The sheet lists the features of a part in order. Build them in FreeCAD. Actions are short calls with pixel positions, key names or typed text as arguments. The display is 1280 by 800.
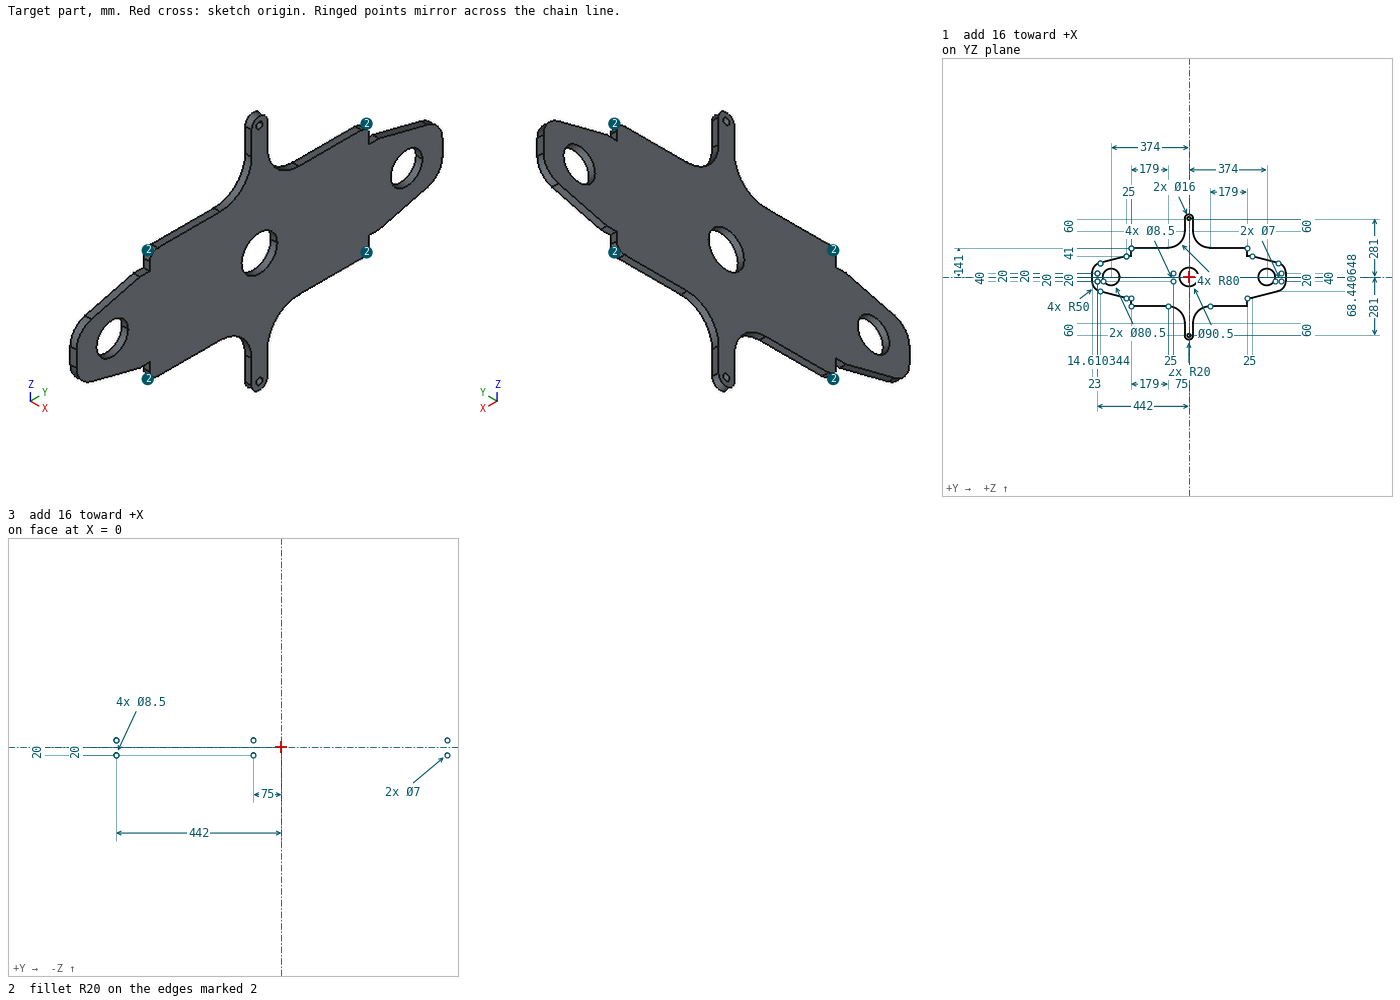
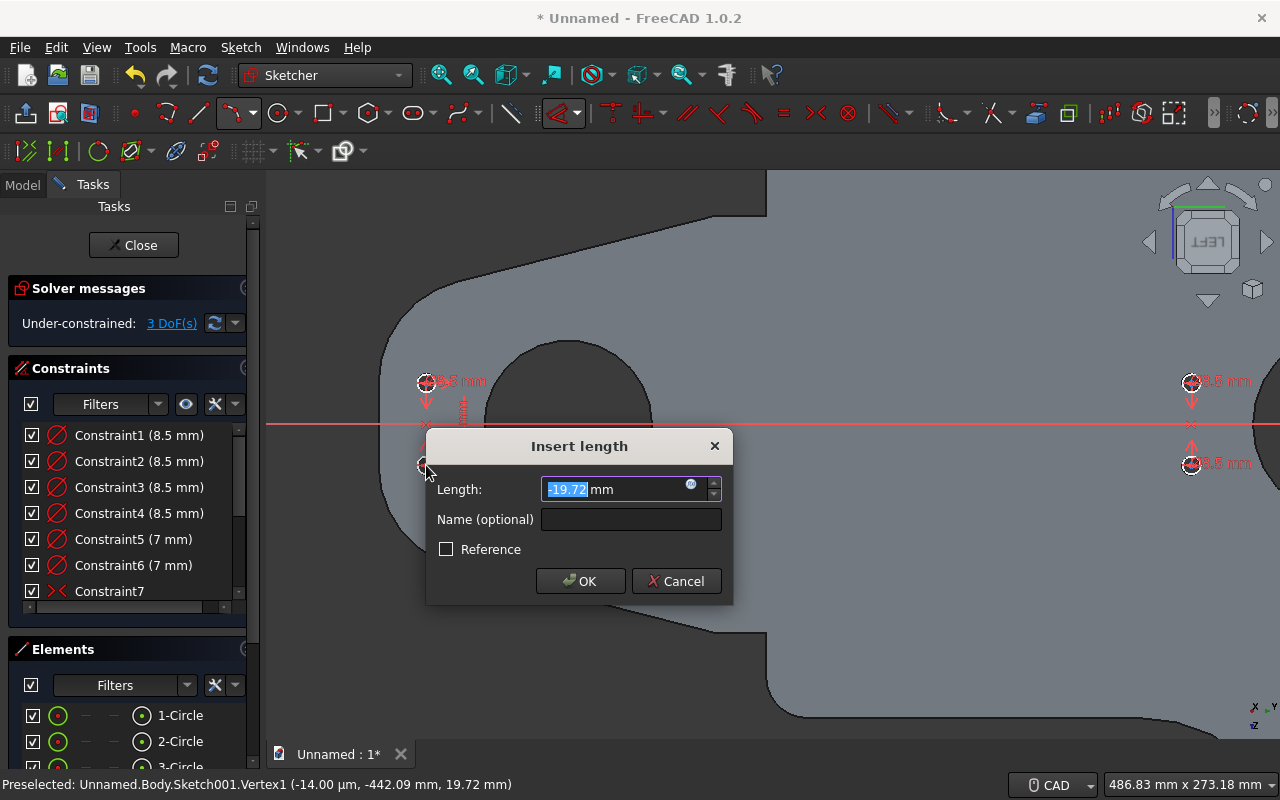
text(-20)
key(Return)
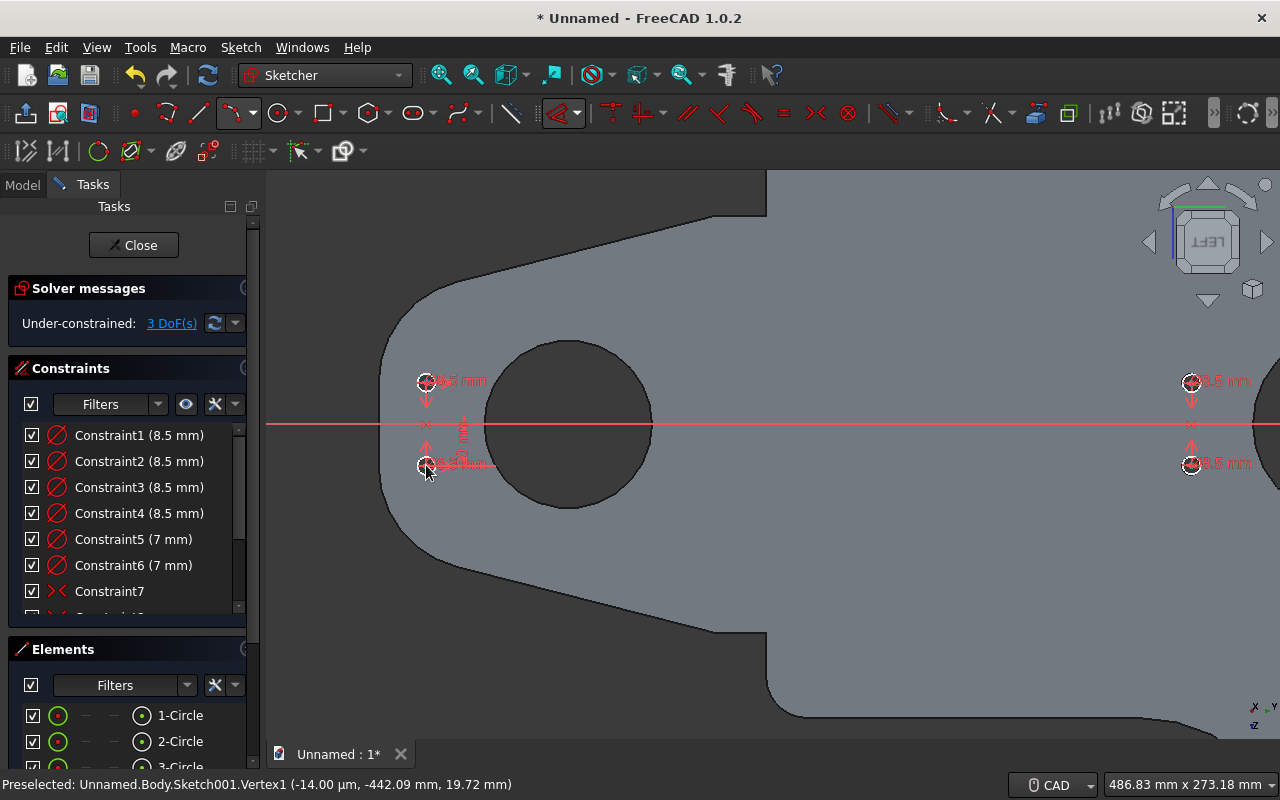
scroll(428, 467, down, 6)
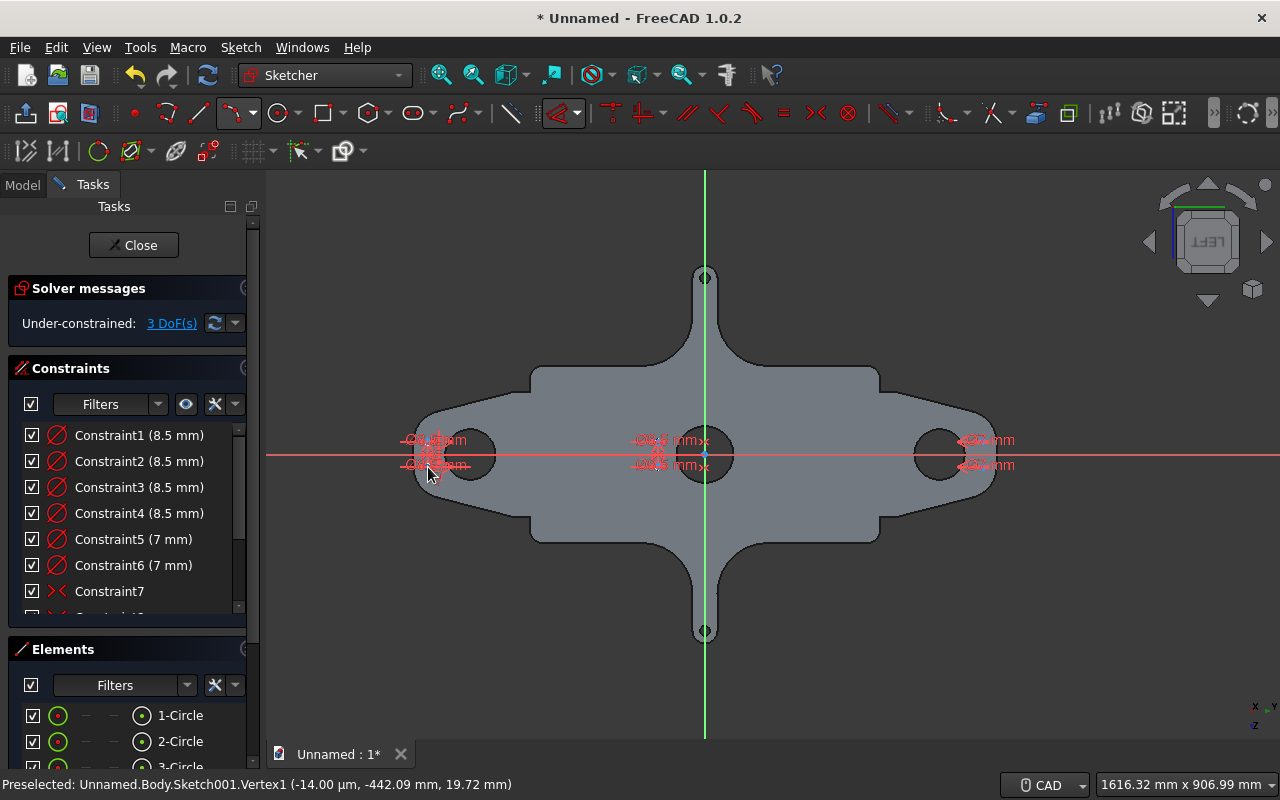
click(658, 467)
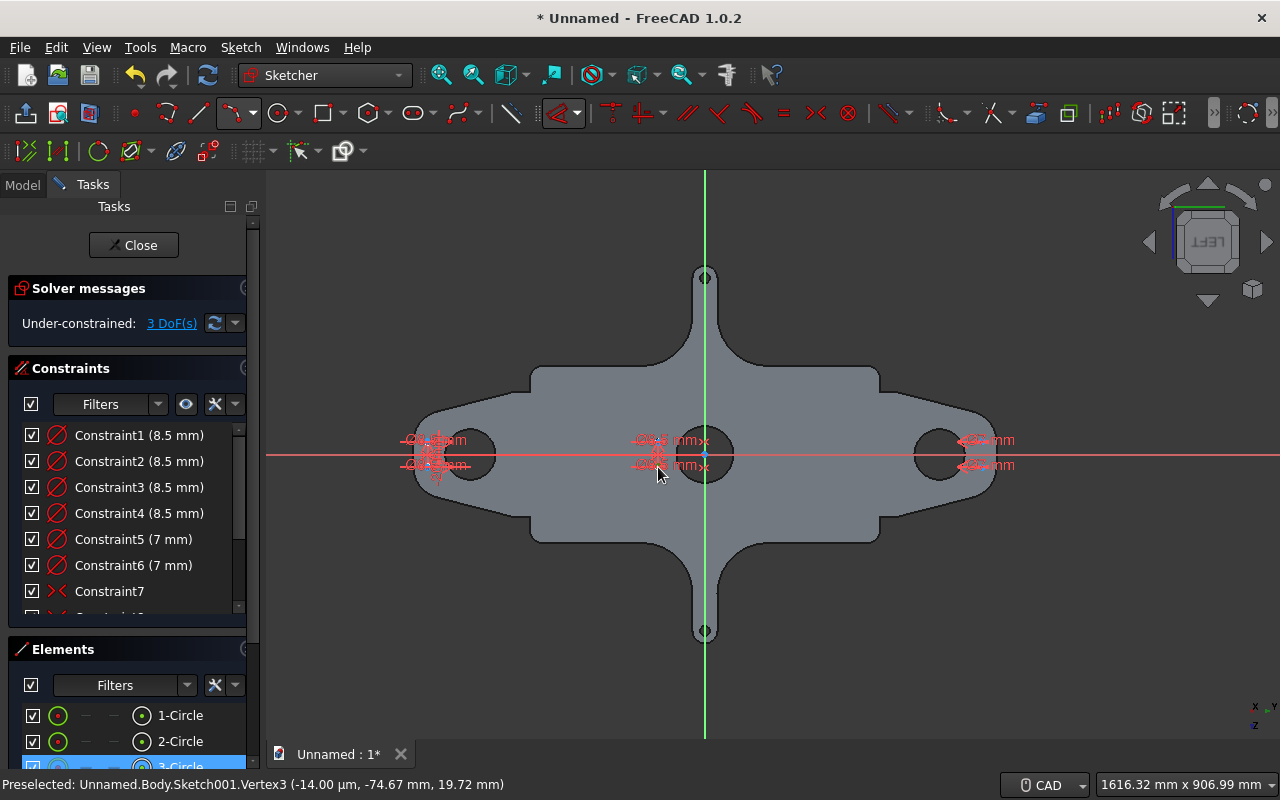
key(l)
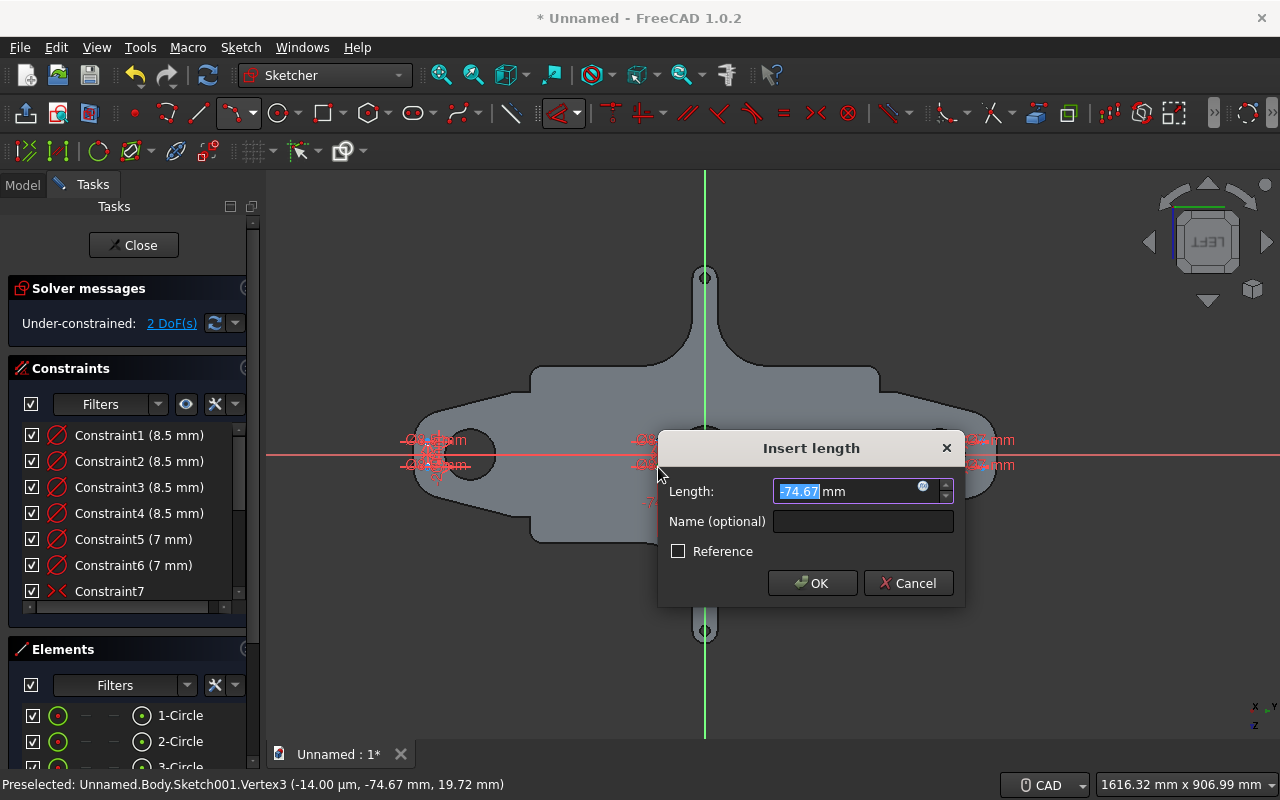
text(-75)
key(Return)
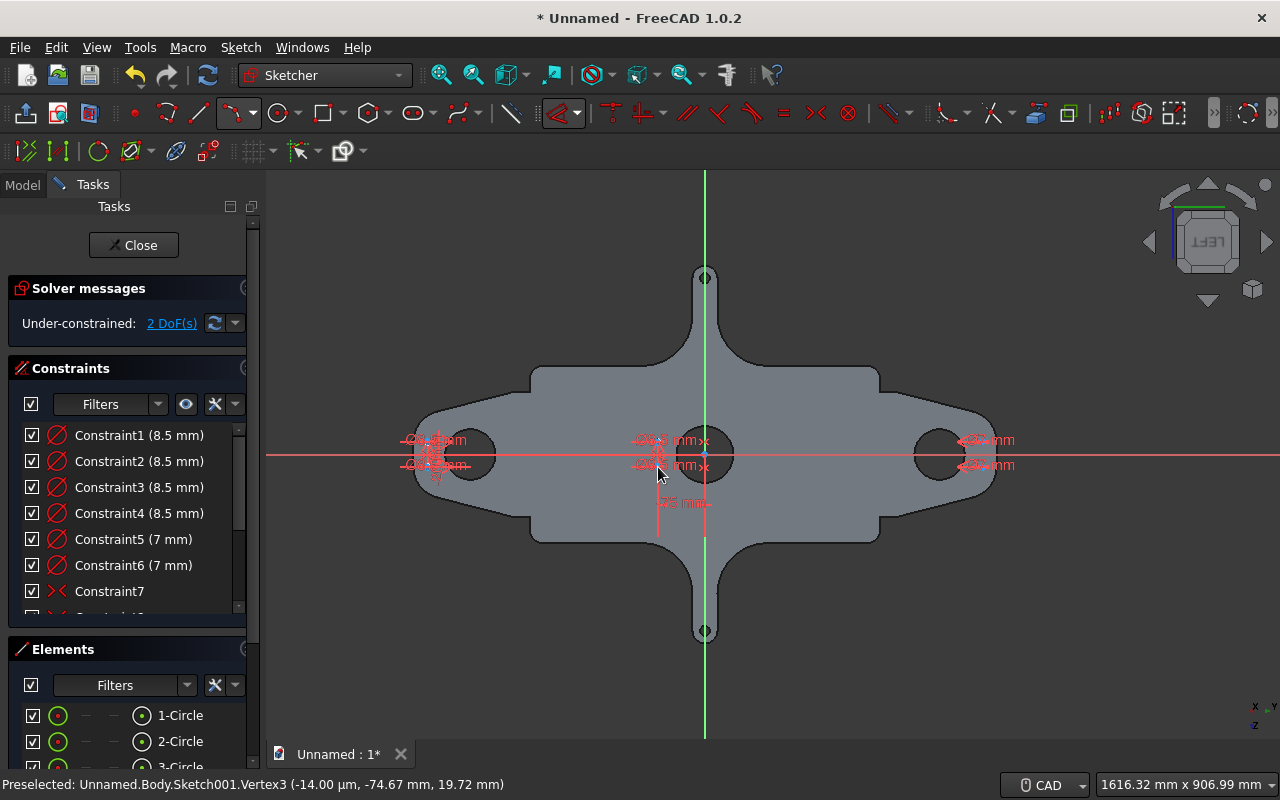
scroll(658, 467, up, 6)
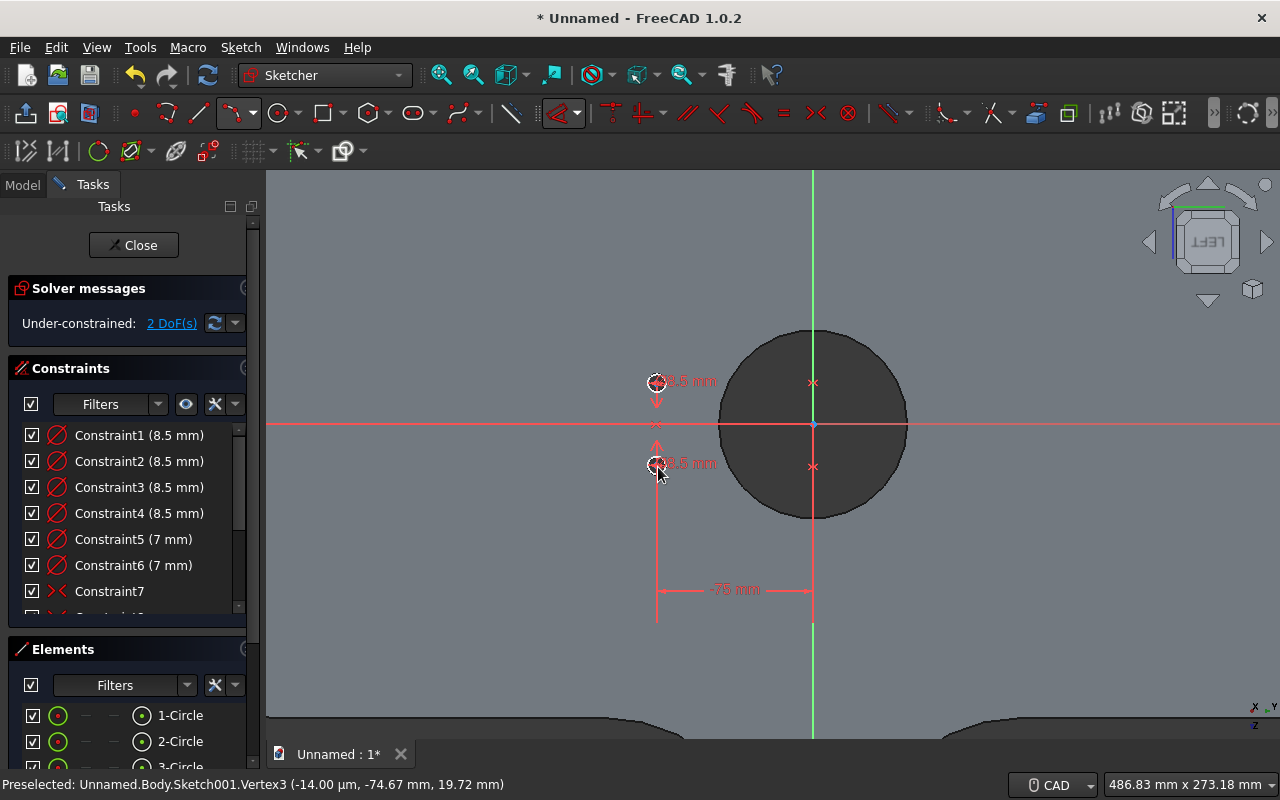
click(657, 465)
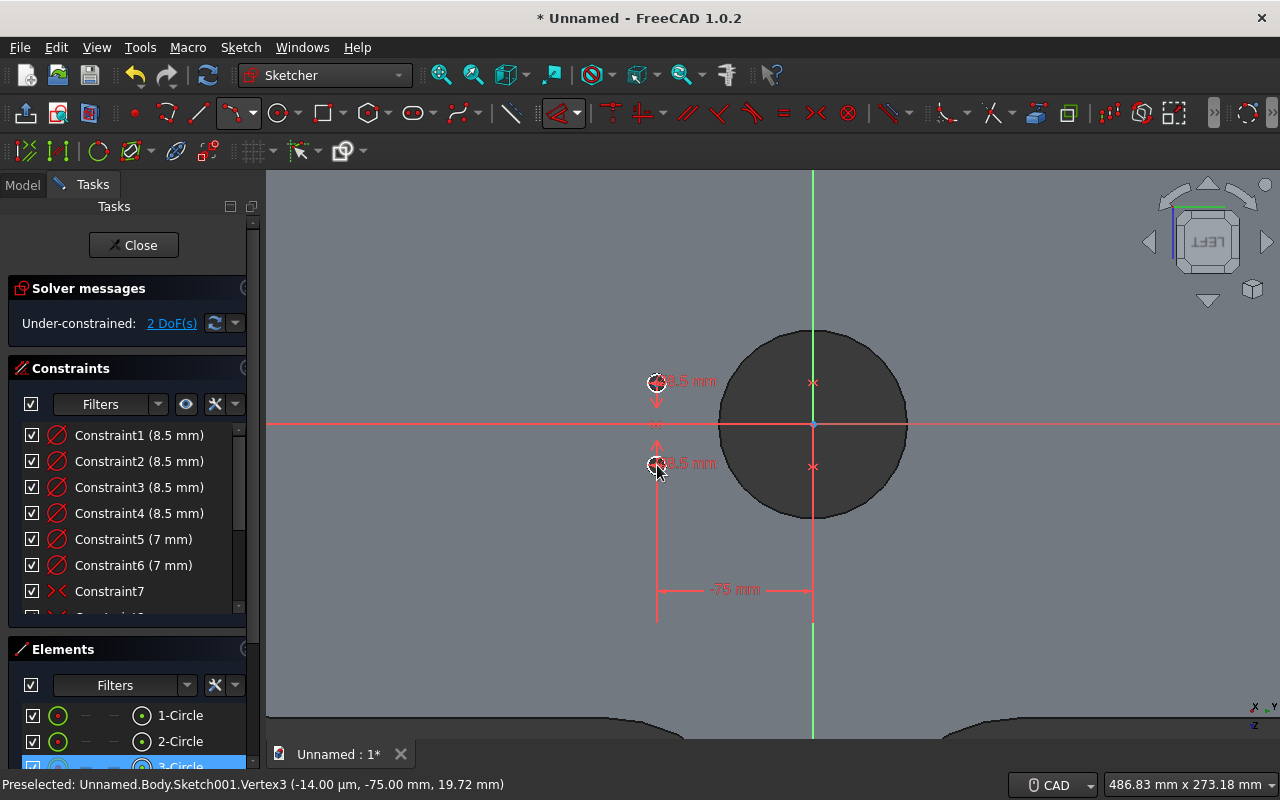
click(580, 114)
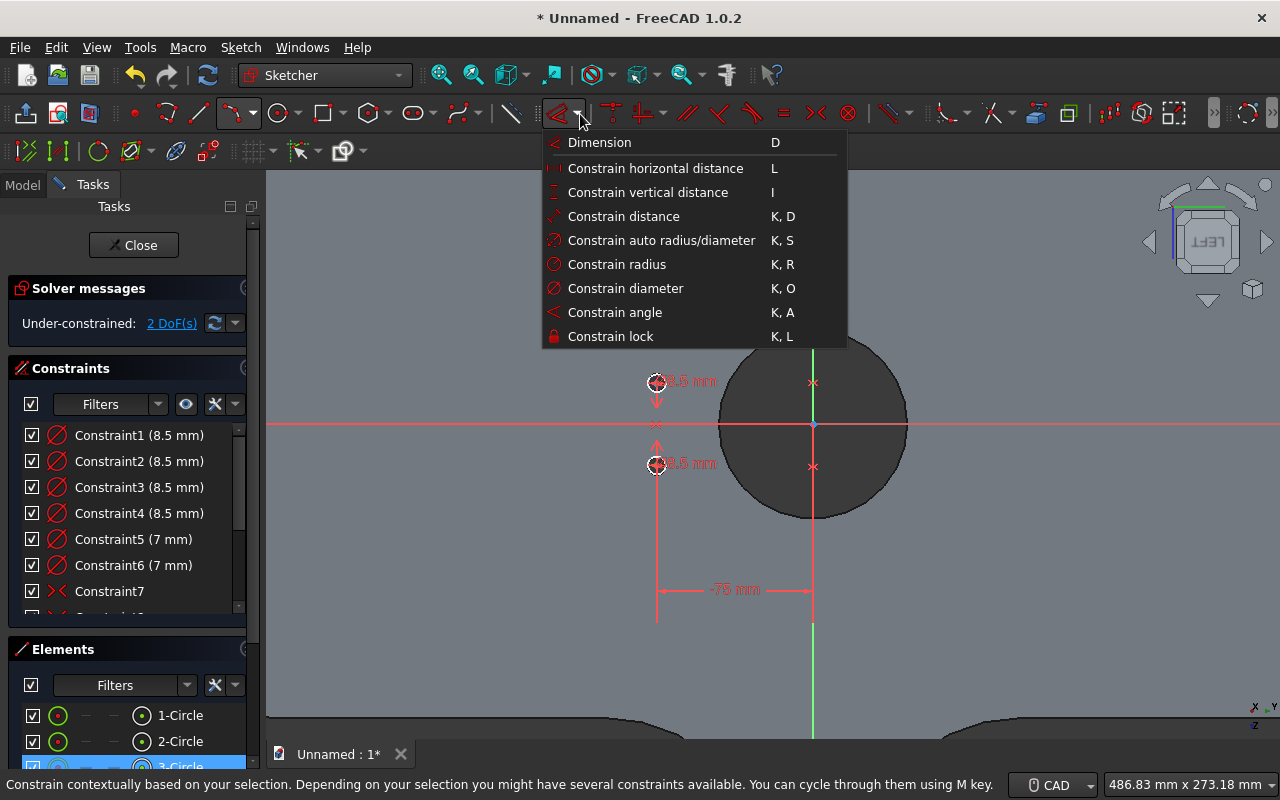
click(695, 192)